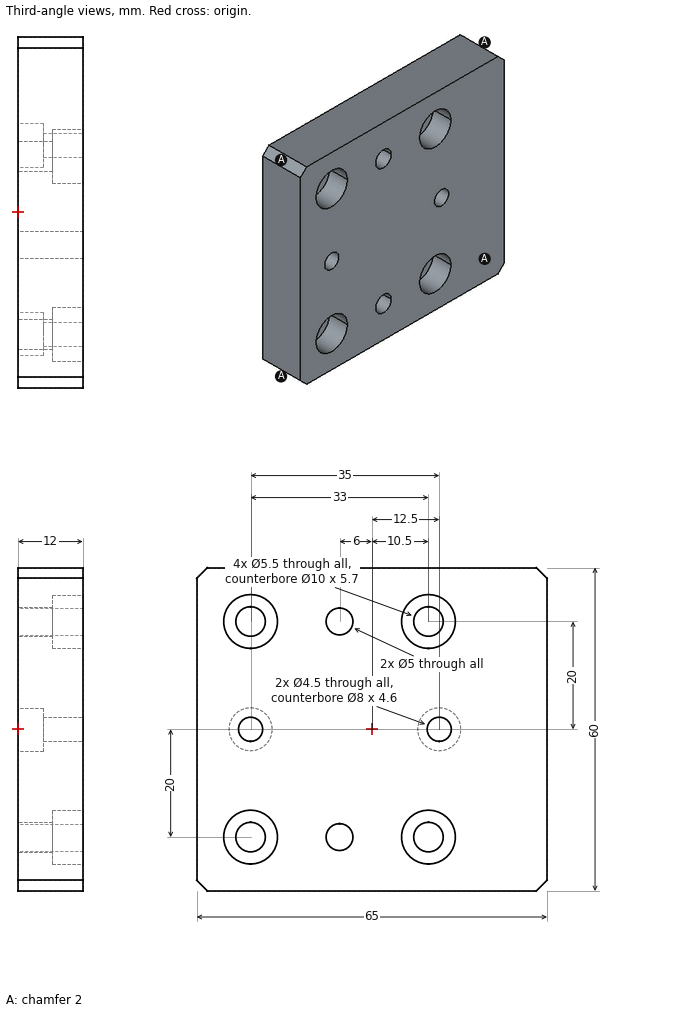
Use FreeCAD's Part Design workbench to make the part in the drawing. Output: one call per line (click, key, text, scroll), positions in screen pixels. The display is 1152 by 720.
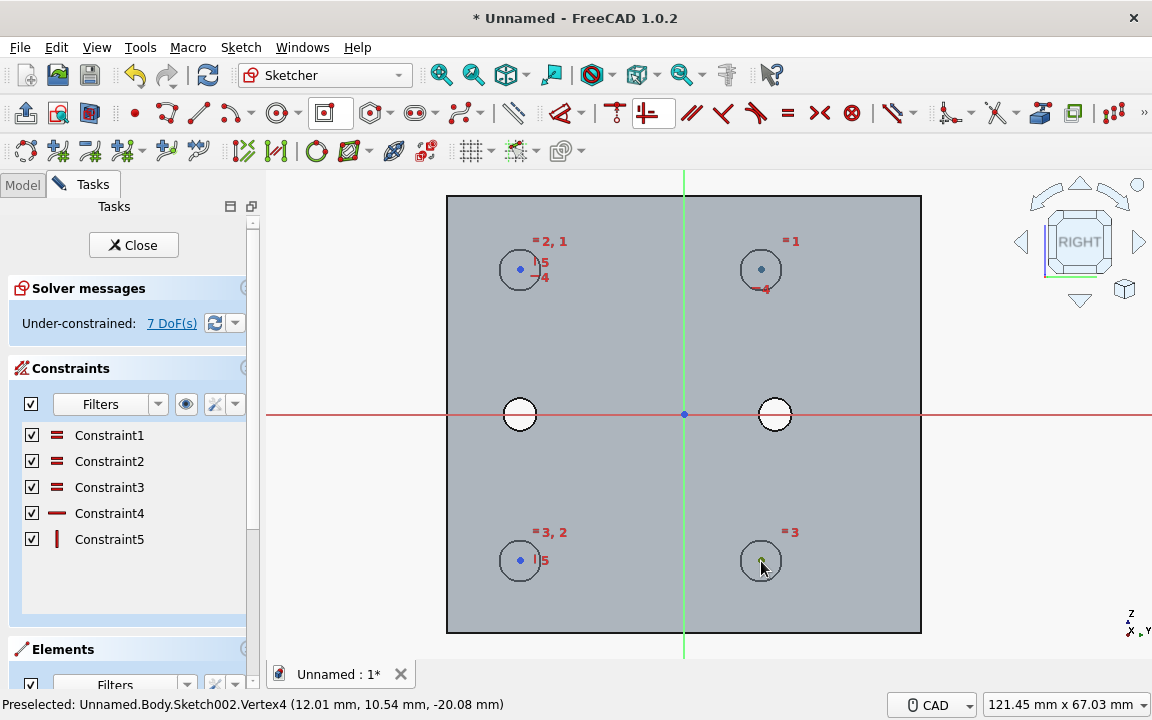
click(670, 114)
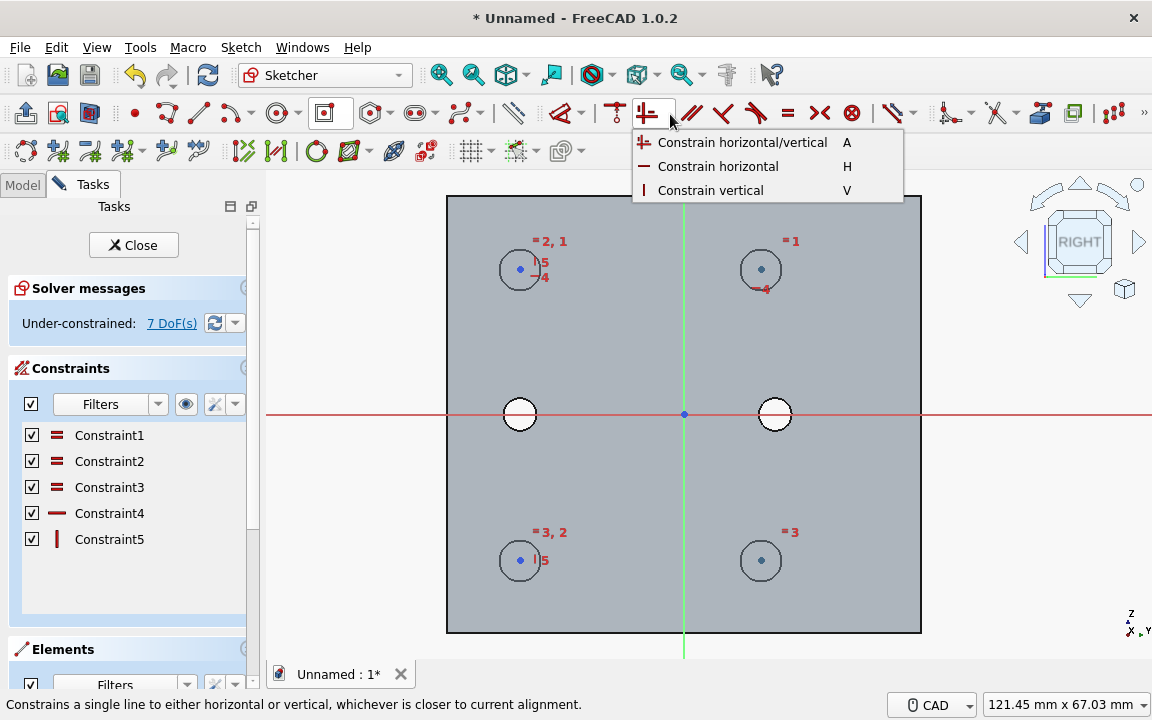
click(768, 190)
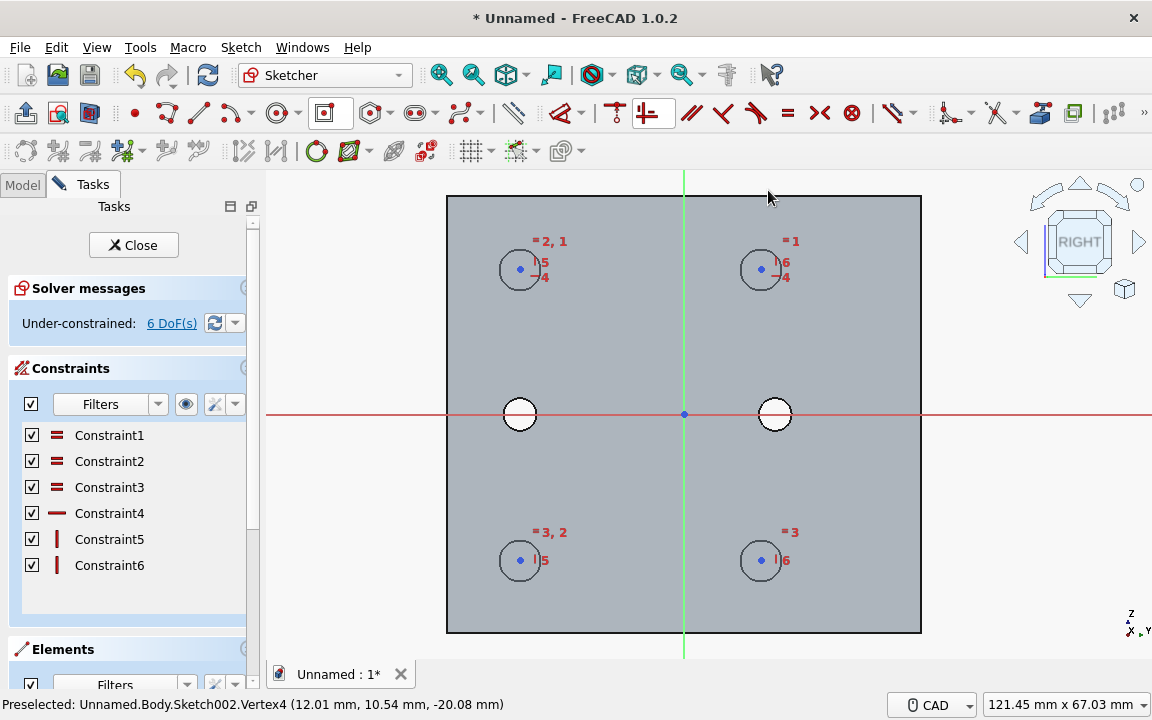
click(520, 561)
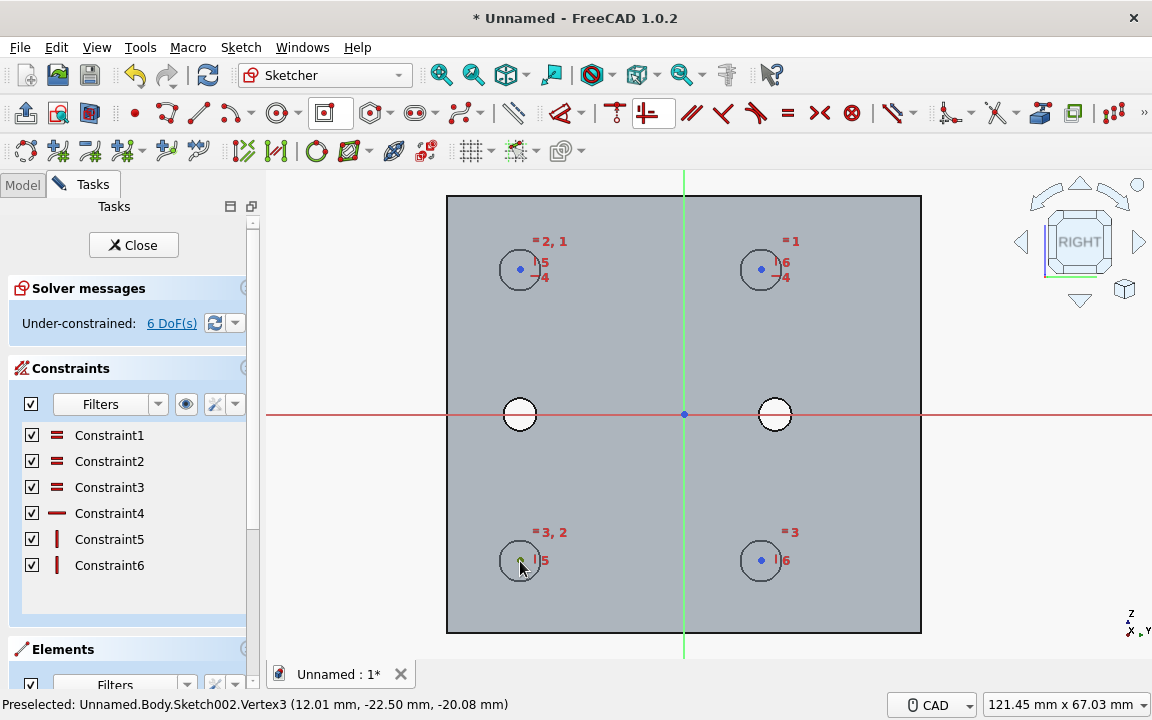
click(761, 561)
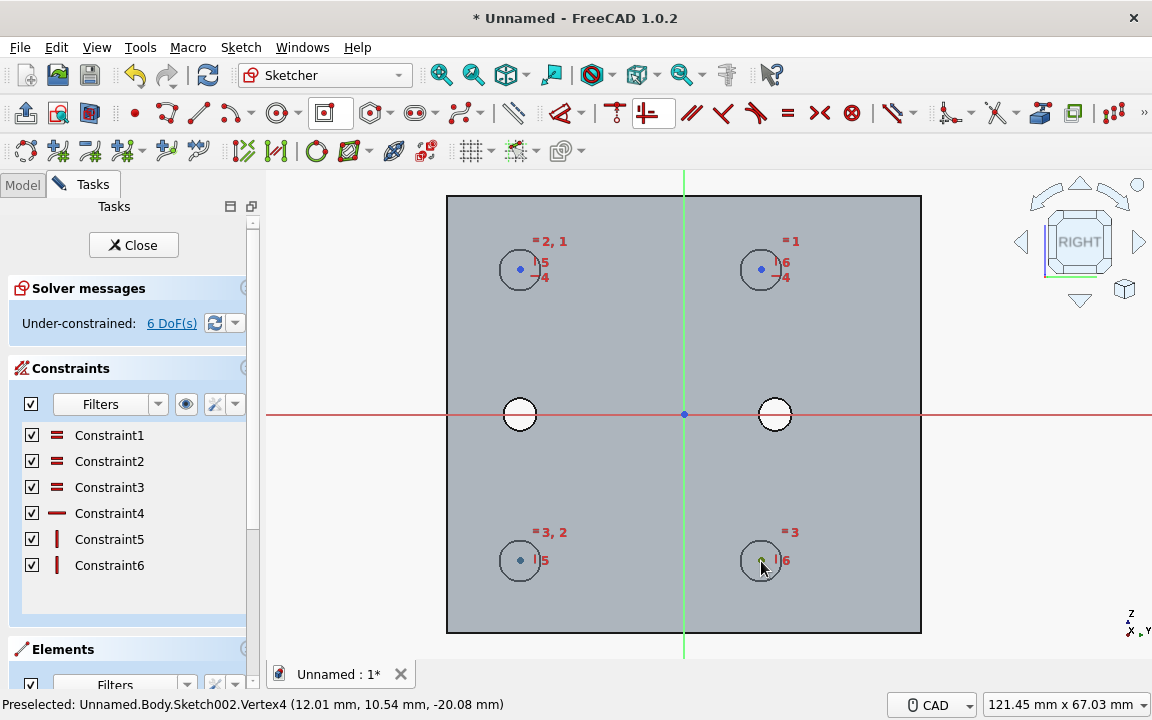
click(670, 114)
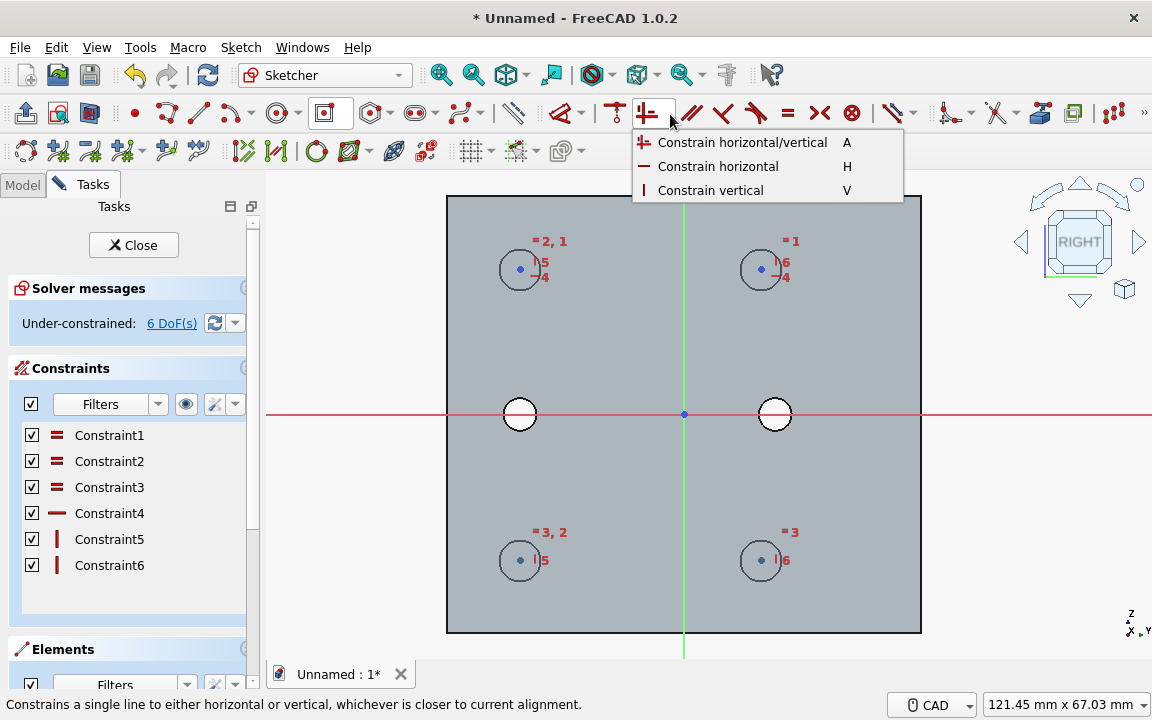
click(768, 166)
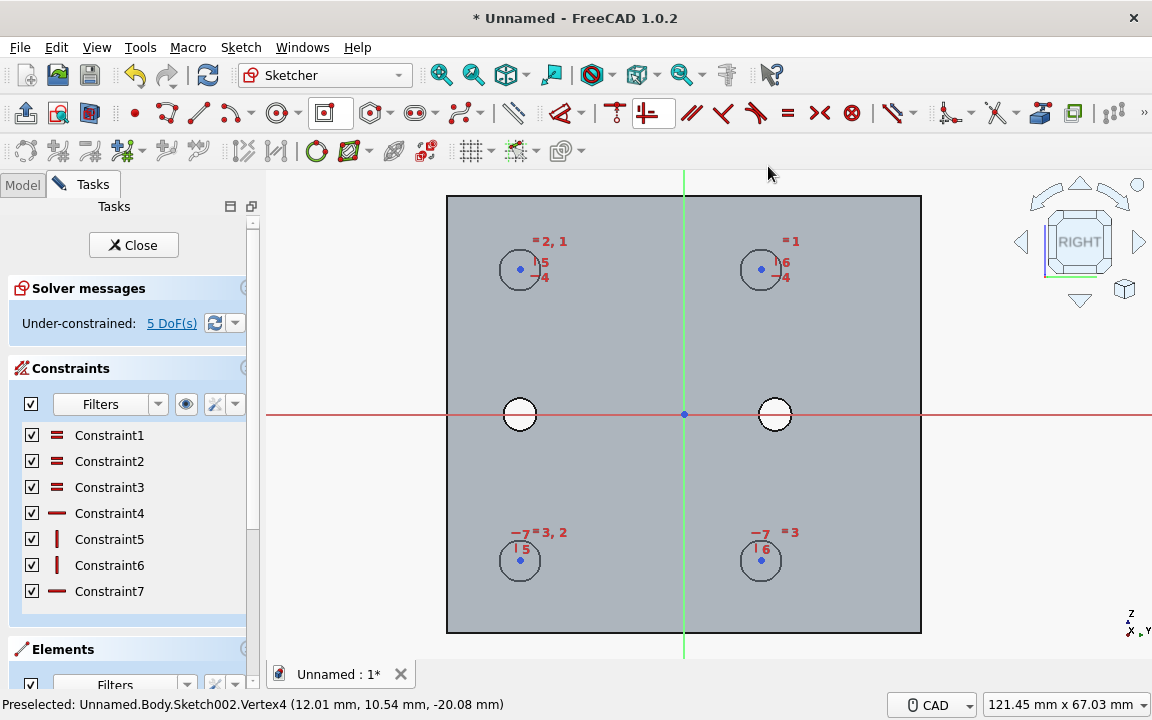
click(560, 114)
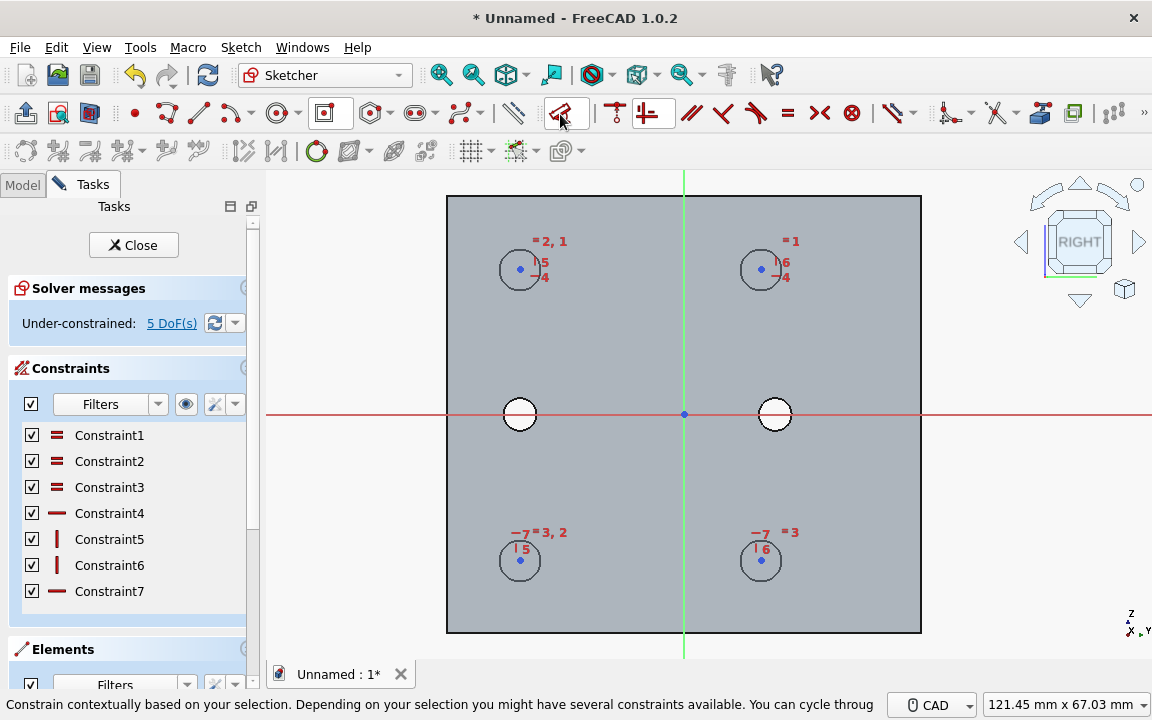
click(775, 255)
click(797, 232)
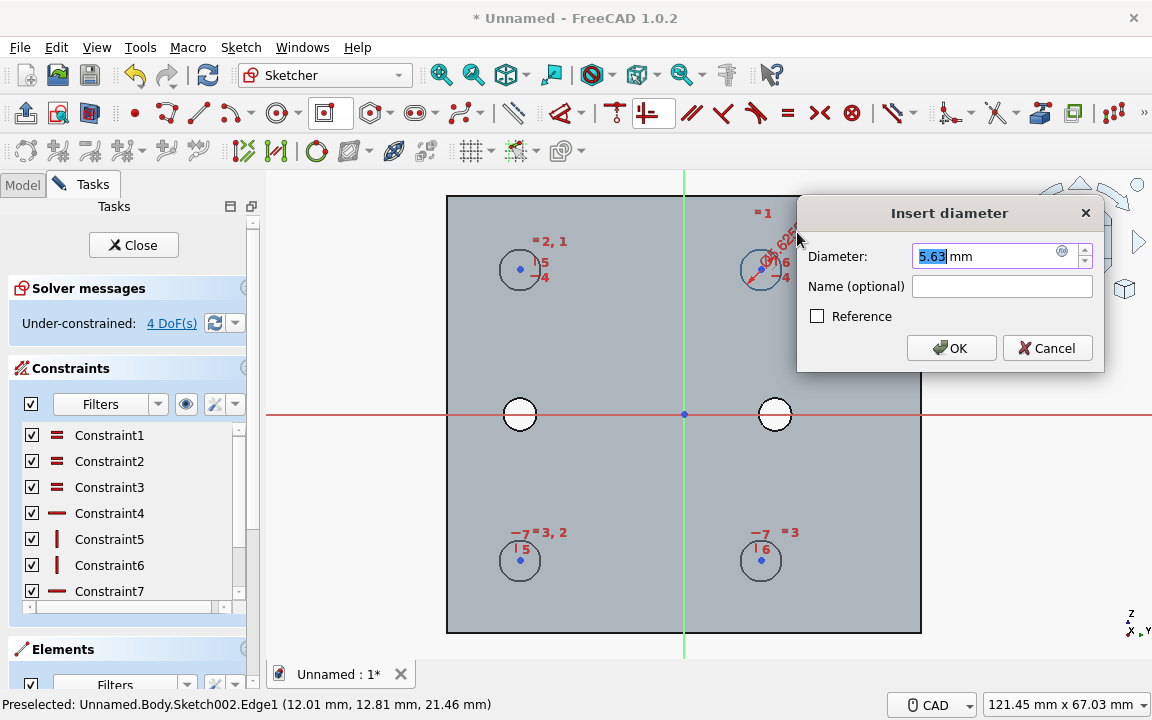
text(5.5)
key(Return)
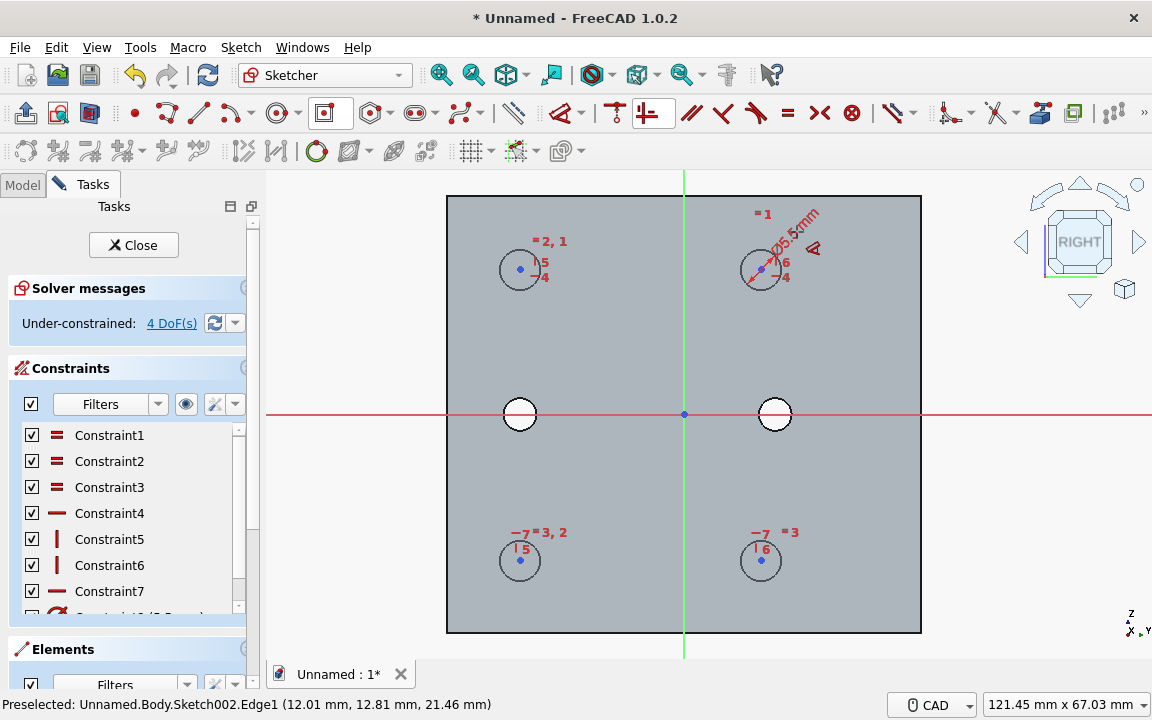
click(761, 270)
click(795, 342)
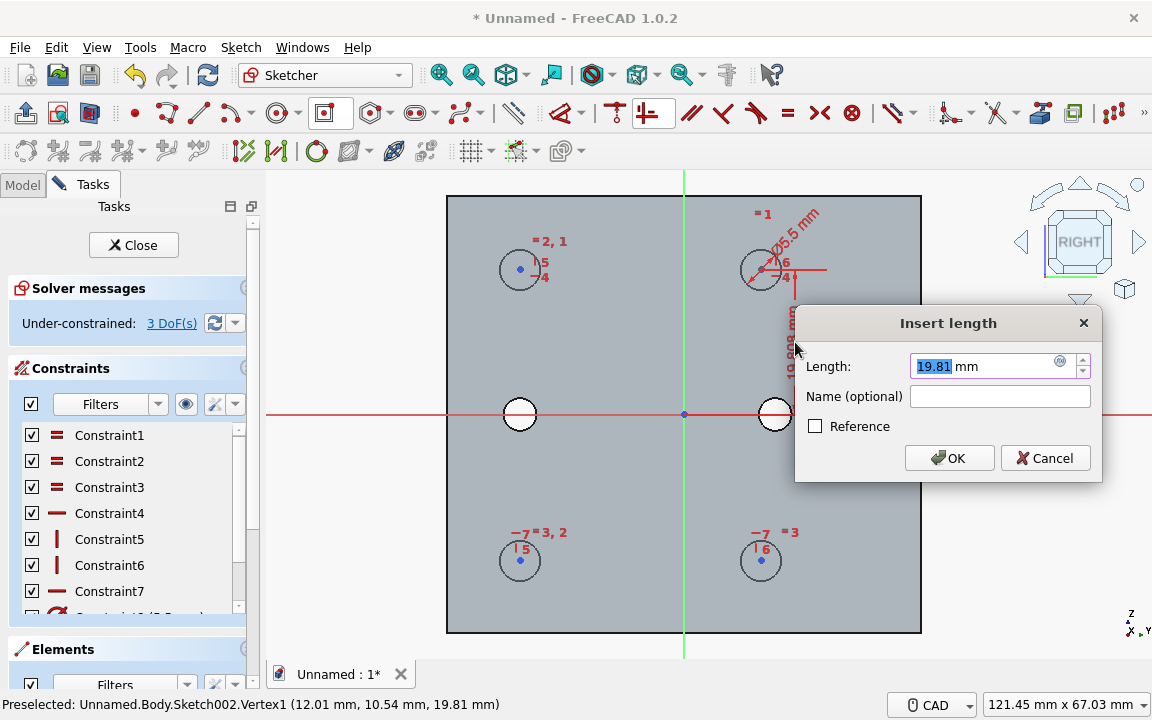
text(20)
key(Return)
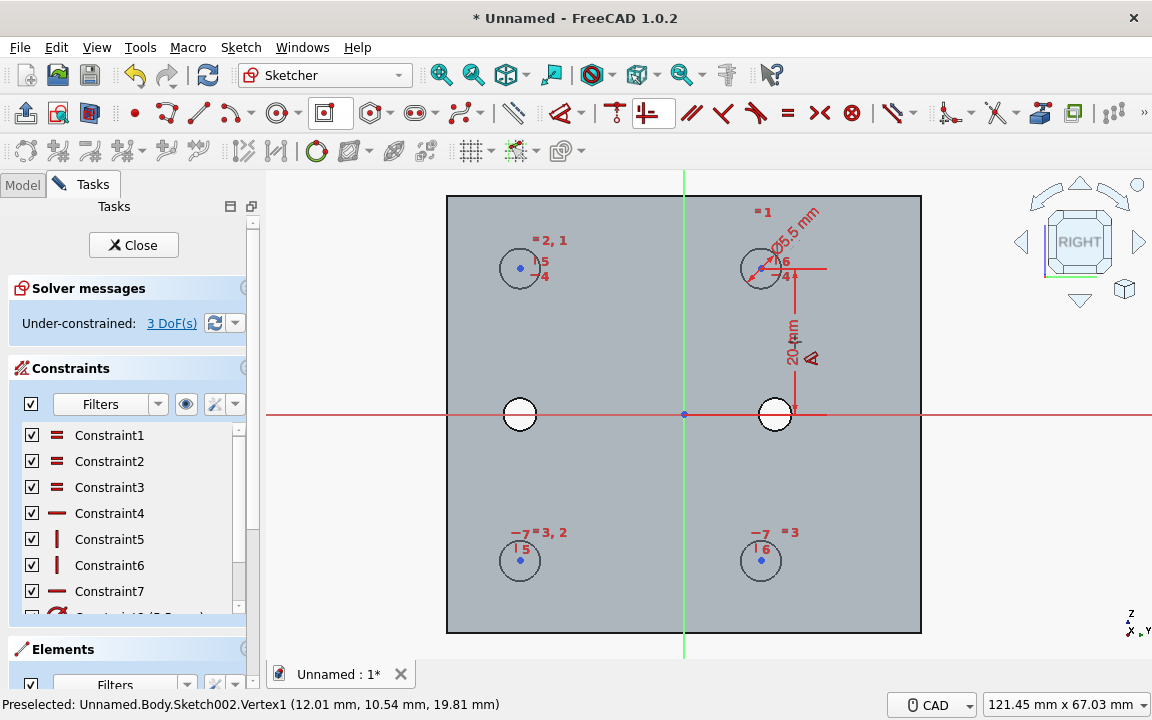
click(520, 561)
click(486, 488)